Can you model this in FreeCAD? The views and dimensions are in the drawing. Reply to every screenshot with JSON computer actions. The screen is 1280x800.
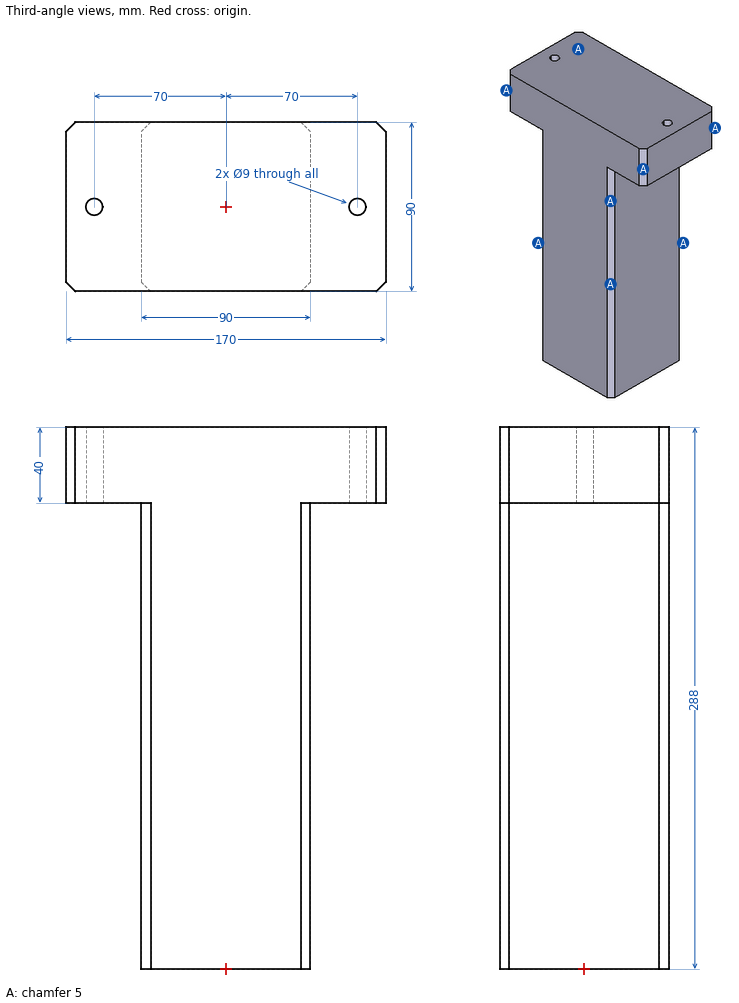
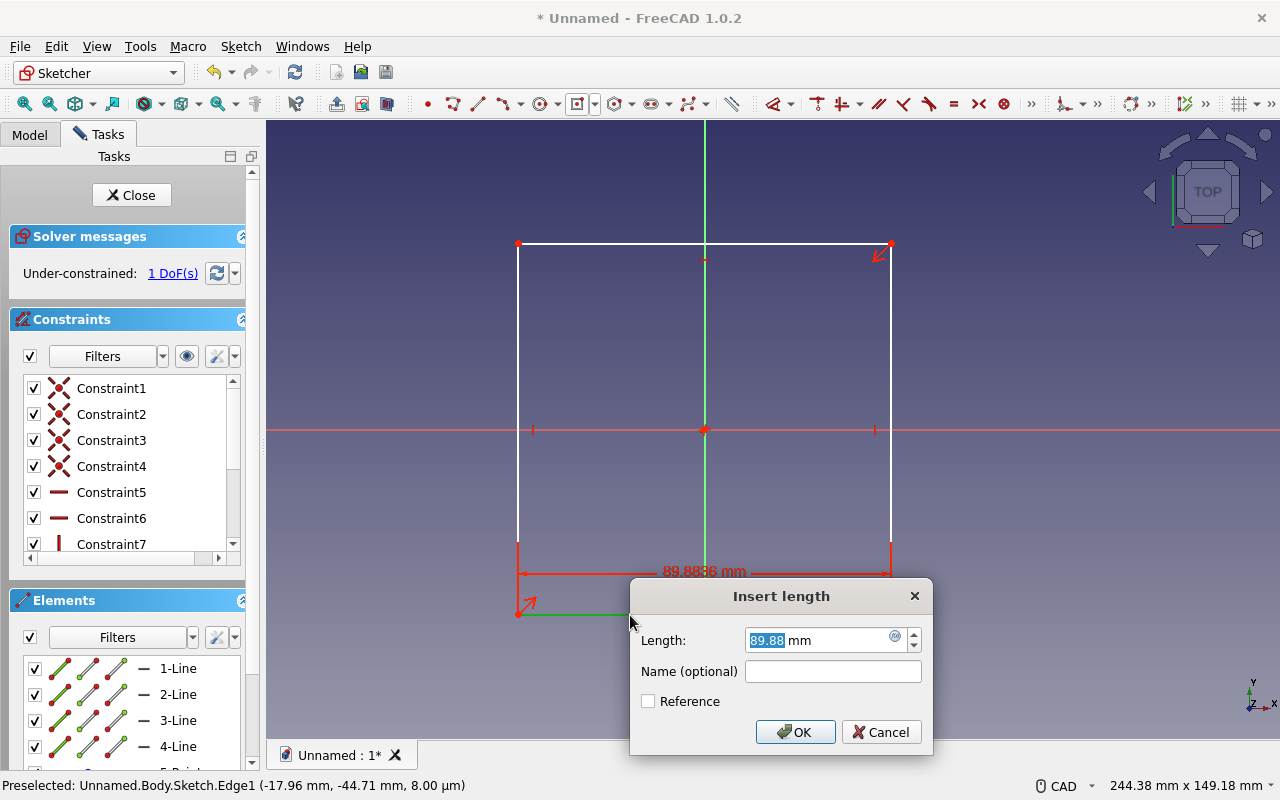
{"action": "type", "text": "90"}
{"action": "key", "text": "Return"}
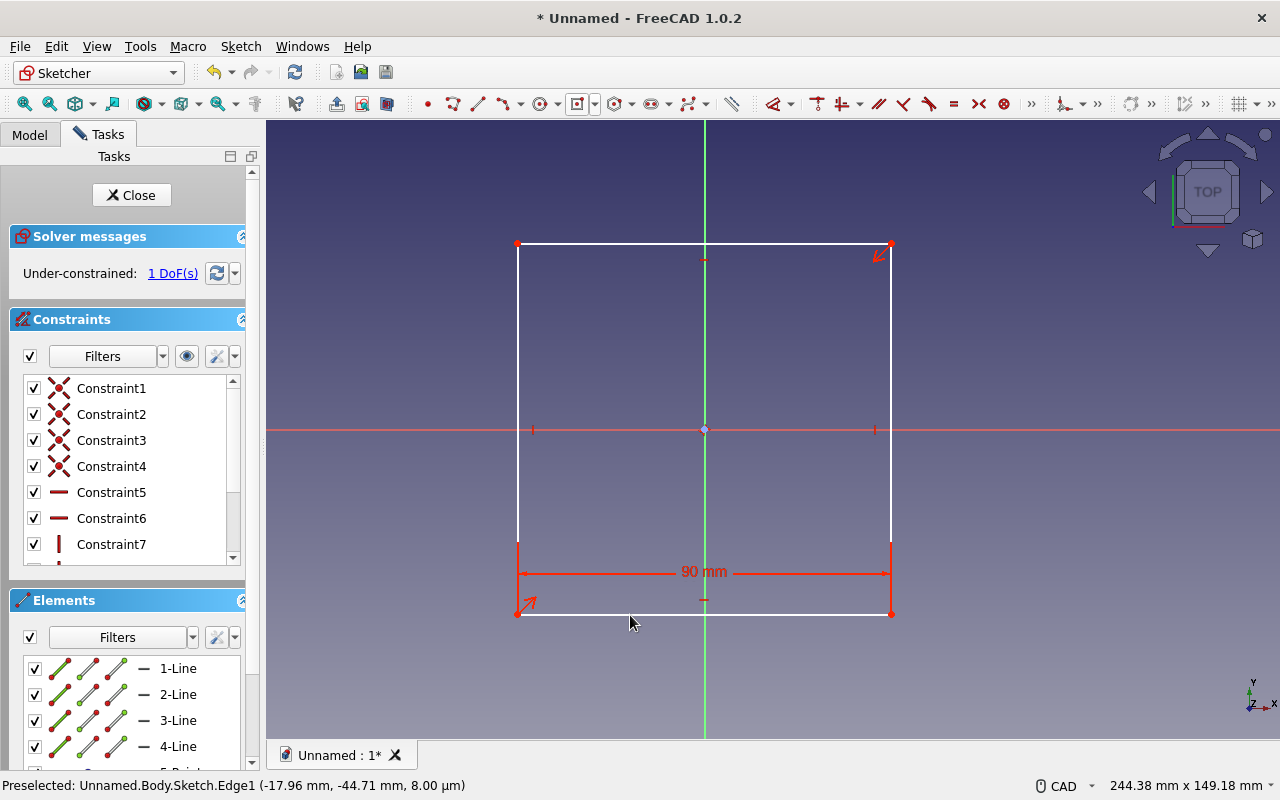
{"action": "left_click", "coordinate": [891, 504]}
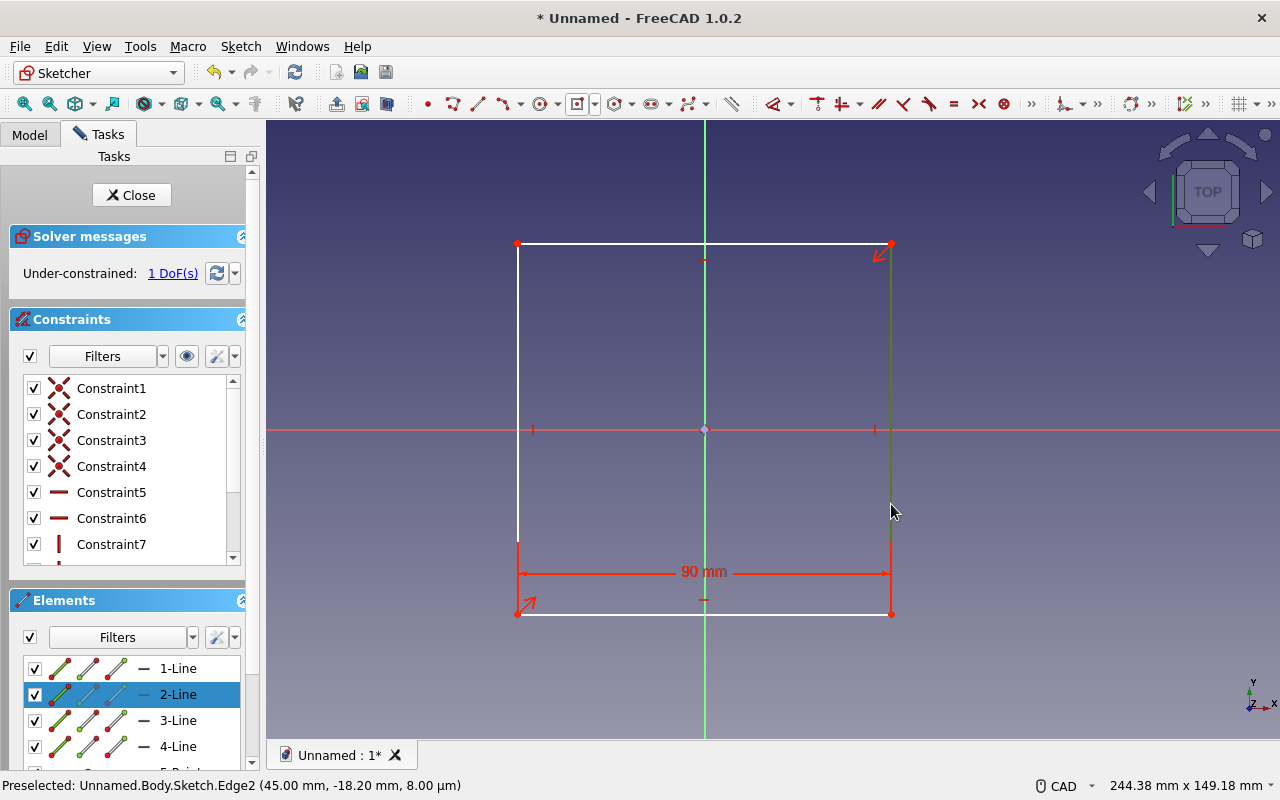
{"action": "key", "text": "i"}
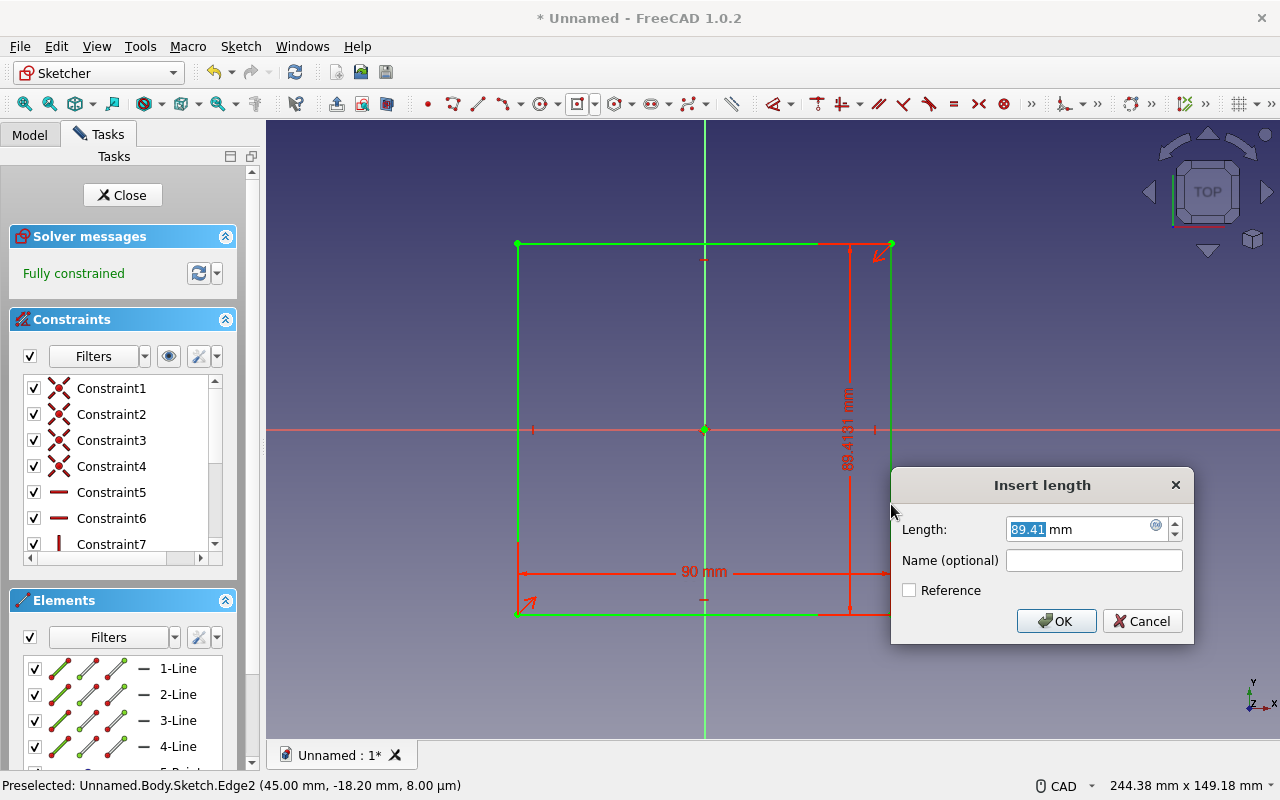
{"action": "type", "text": "90"}
{"action": "key", "text": "Return"}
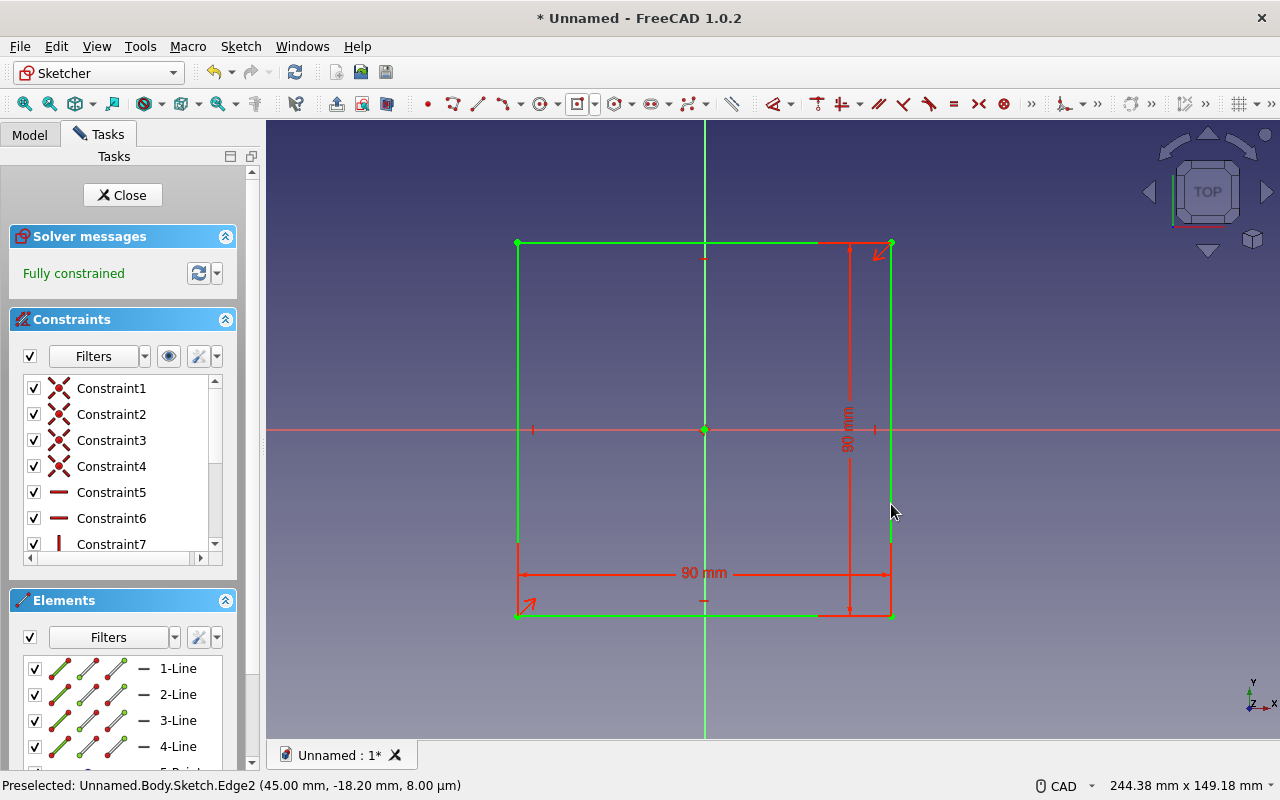
{"action": "left_click", "coordinate": [123, 195]}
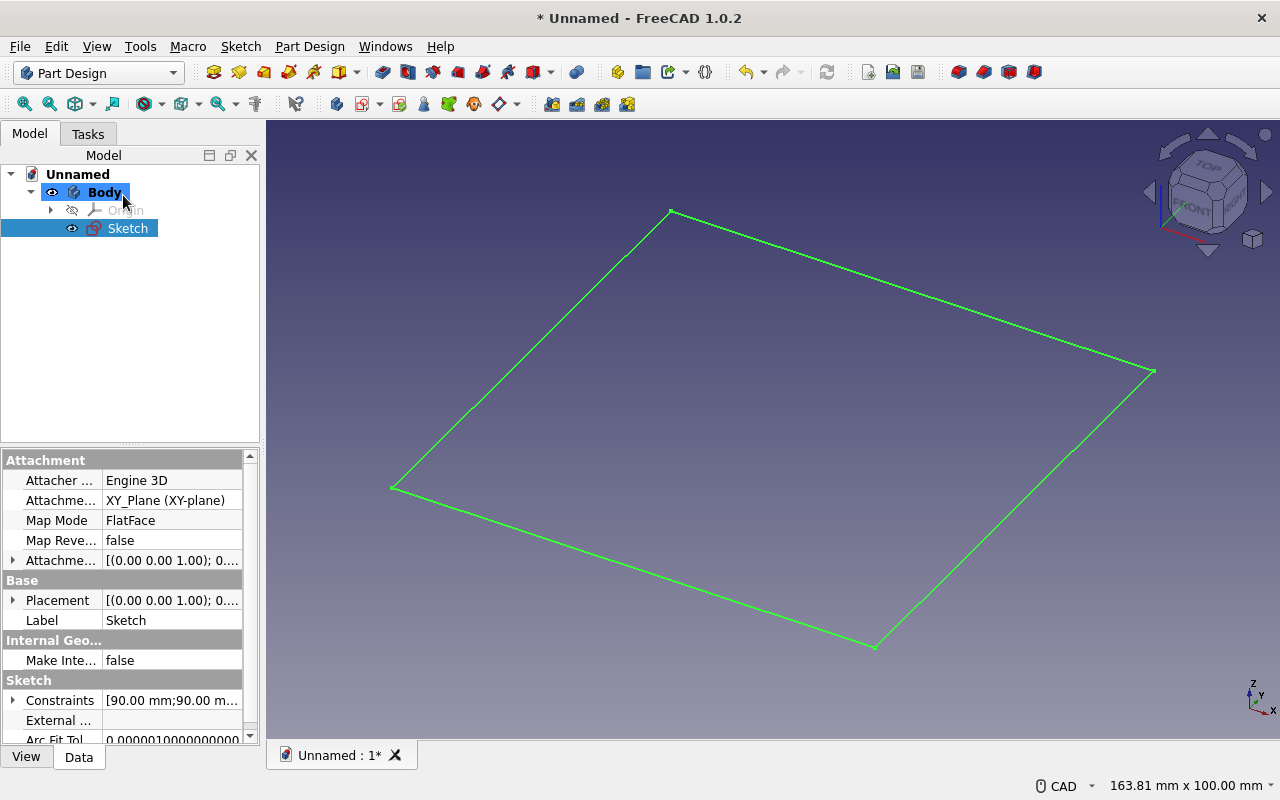
{"action": "left_click", "coordinate": [214, 72]}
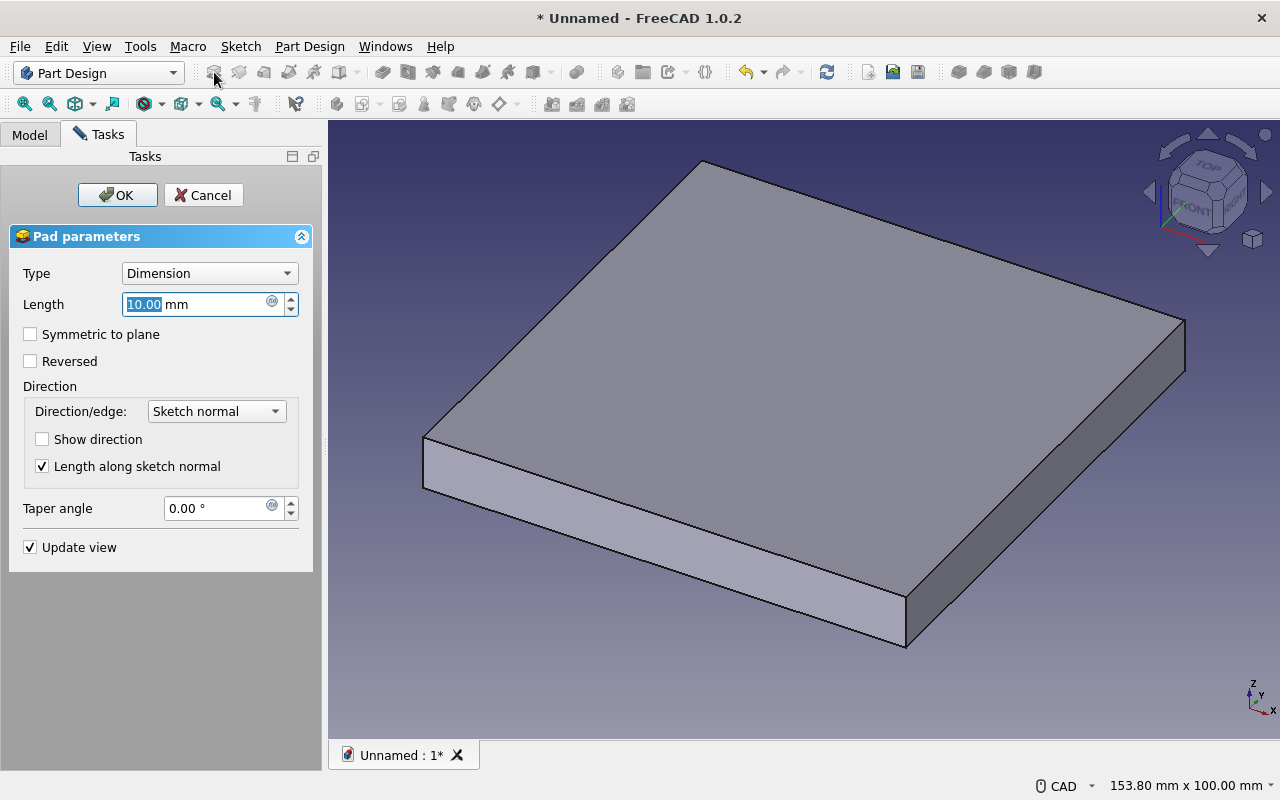
{"action": "type", "text": "288"}
{"action": "key", "text": "Tab"}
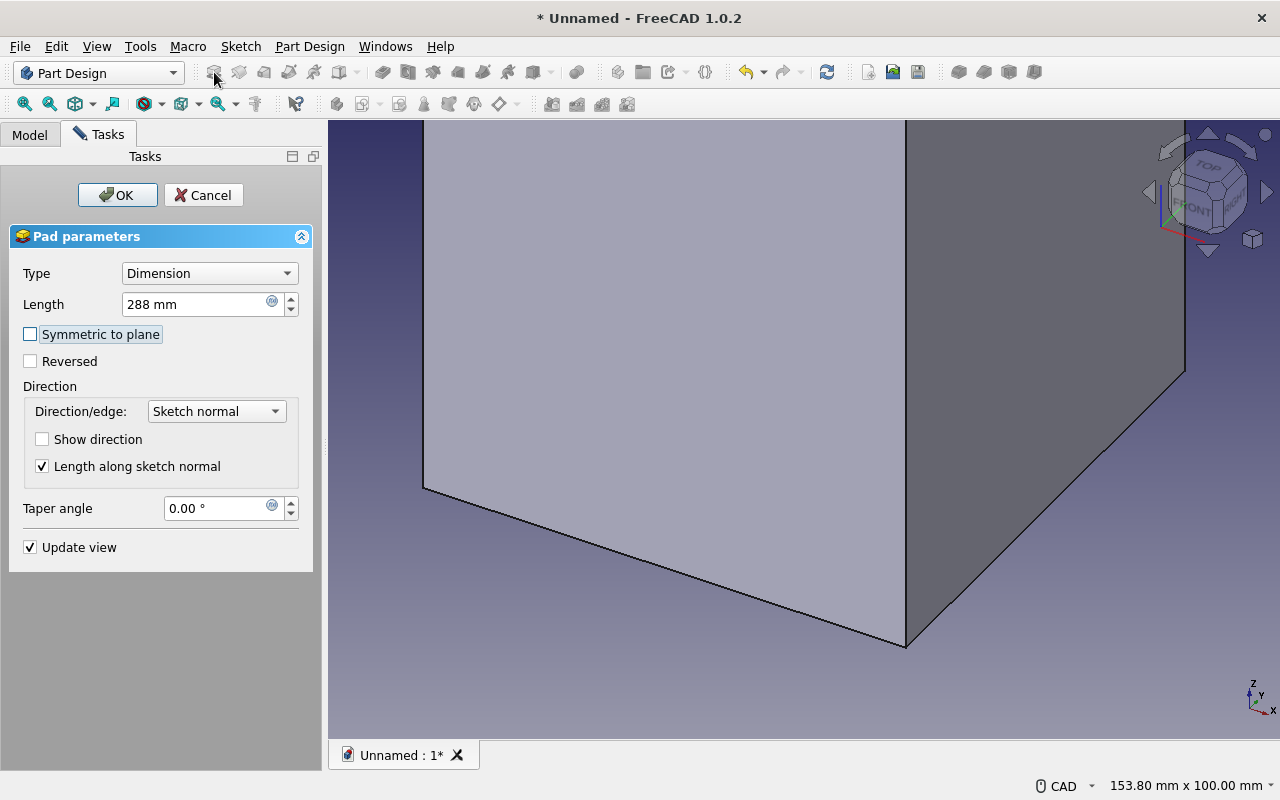
{"action": "left_click", "coordinate": [118, 195]}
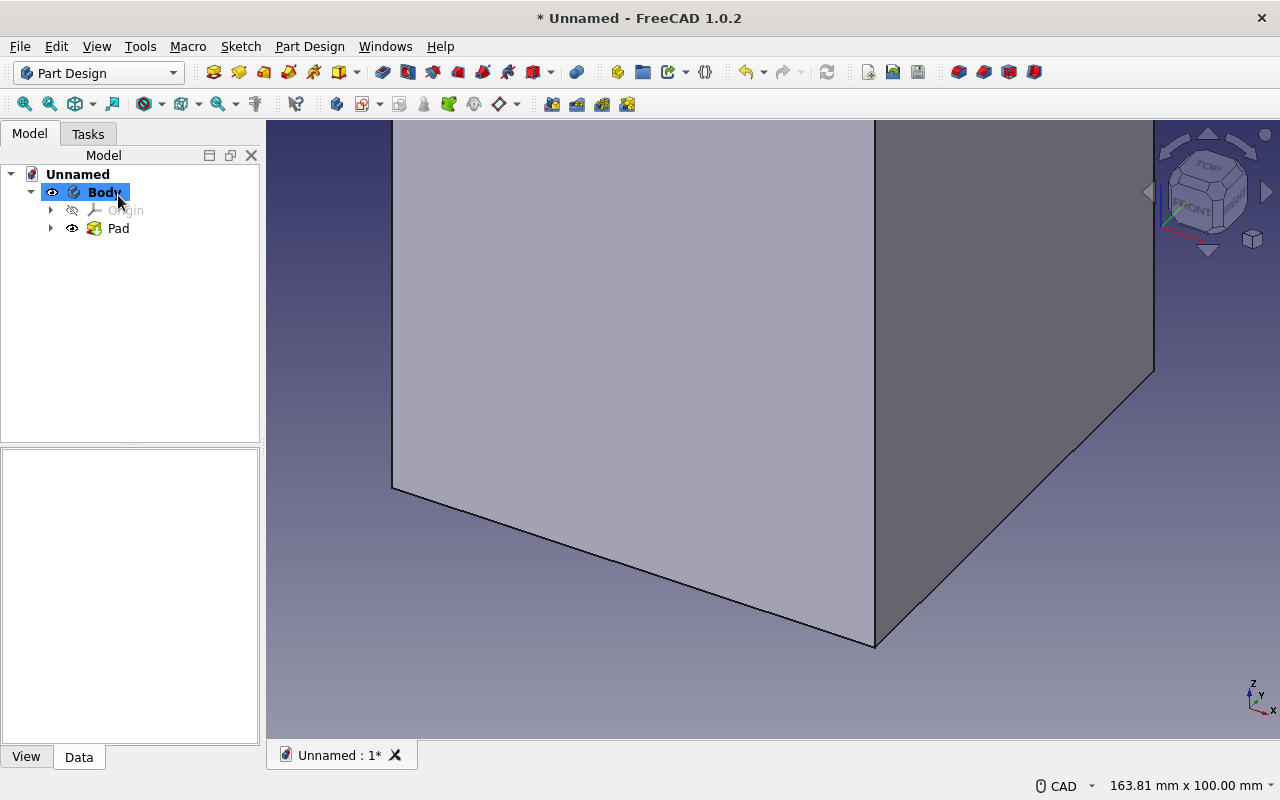
{"action": "left_click", "coordinate": [25, 104]}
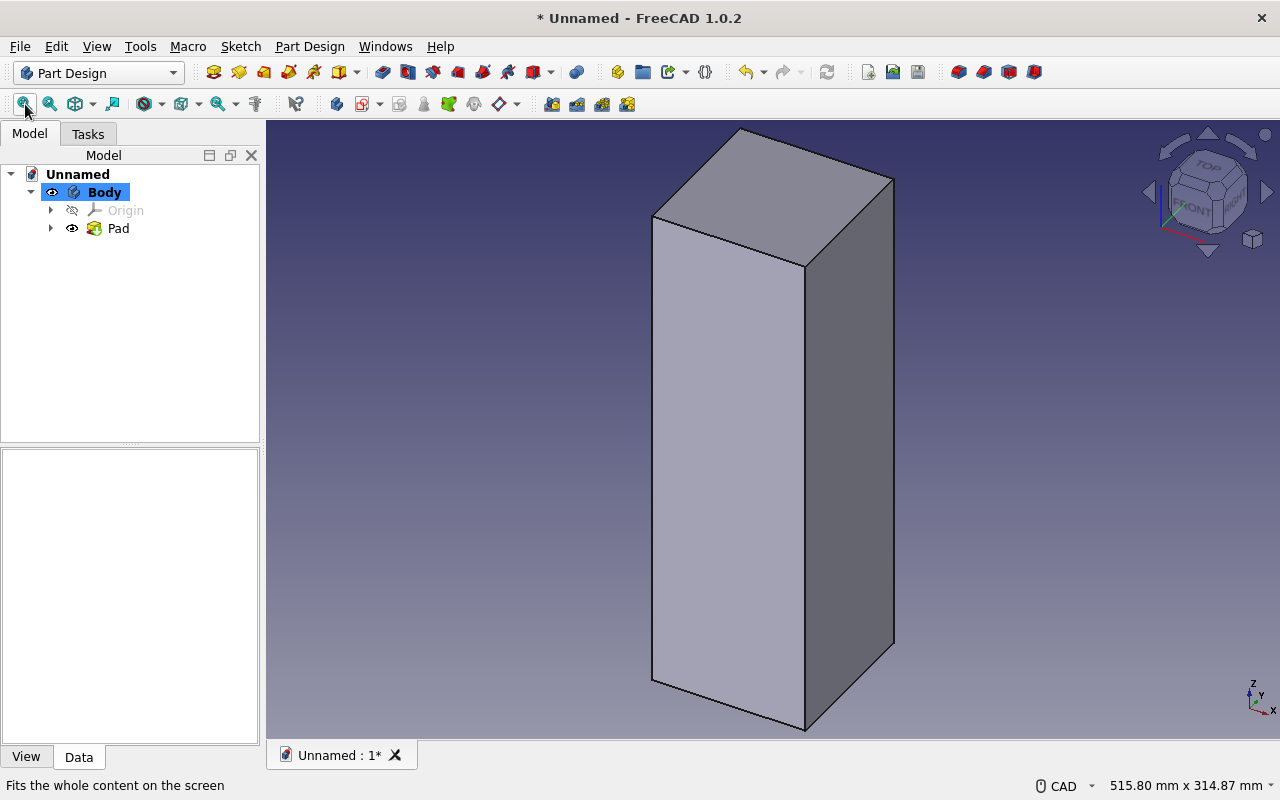
{"action": "left_click", "coordinate": [773, 197]}